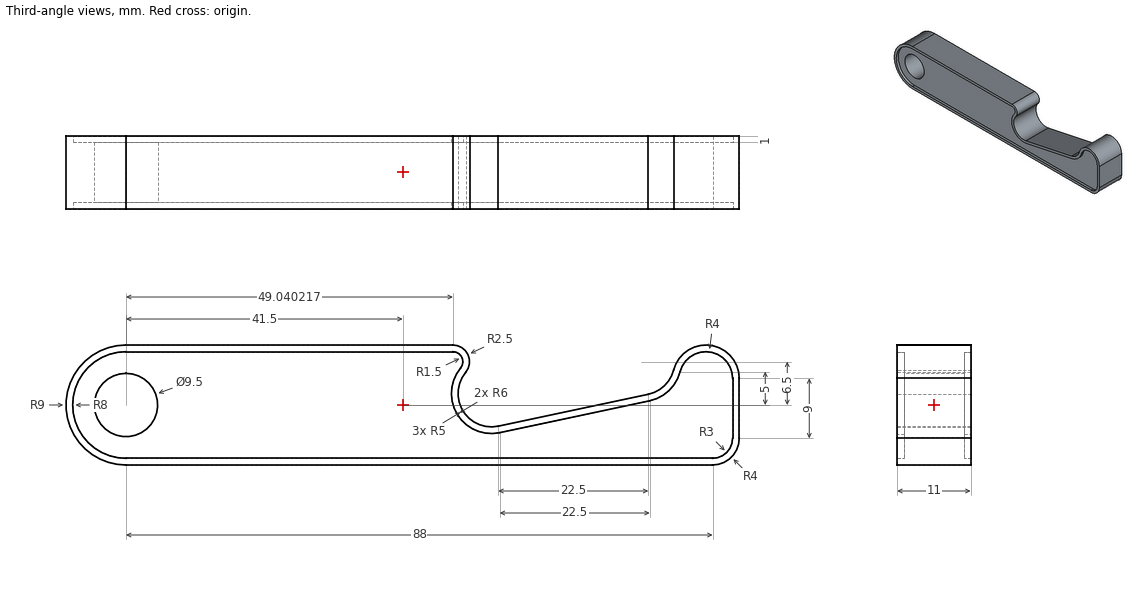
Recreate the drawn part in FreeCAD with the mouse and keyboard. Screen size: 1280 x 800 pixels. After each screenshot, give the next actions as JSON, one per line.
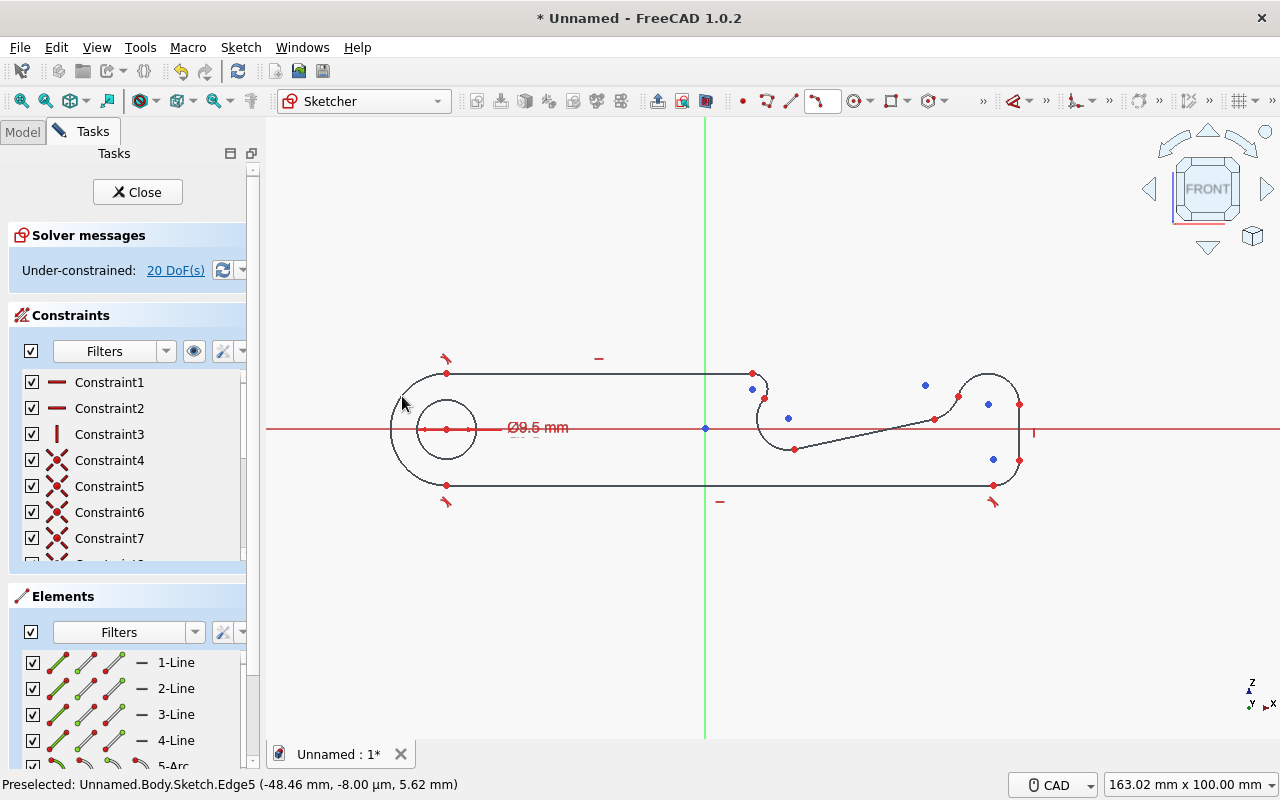
{"action": "left_click", "coordinate": [538, 374]}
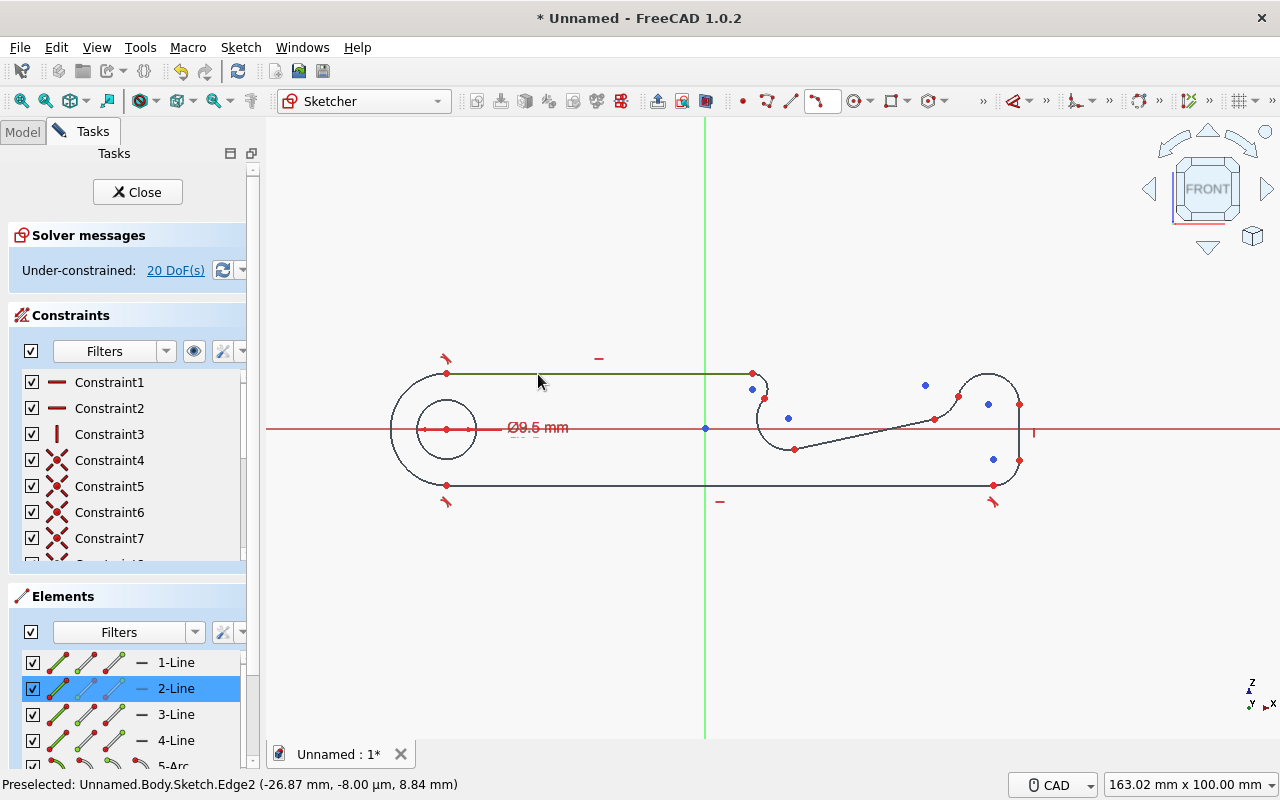
{"action": "scroll", "coordinate": [768, 389], "scroll_direction": "up", "scroll_amount": 2}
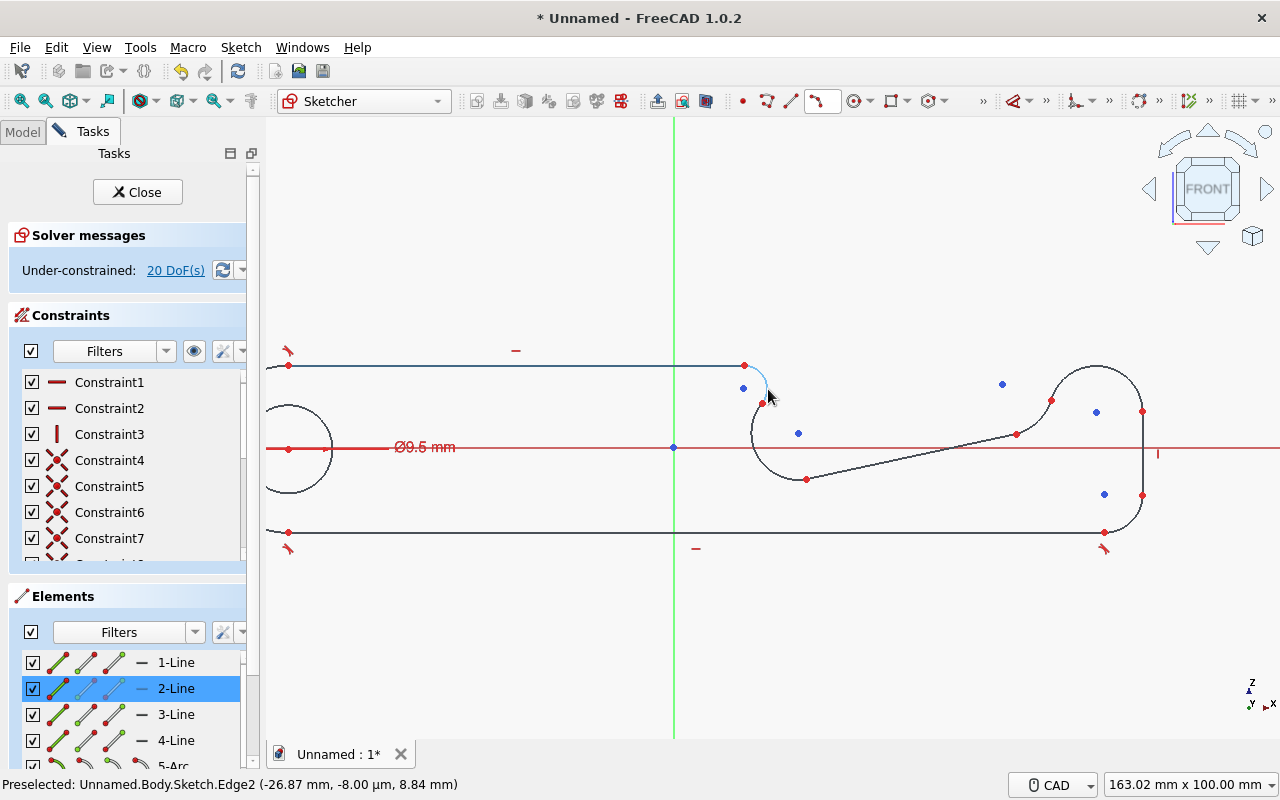
{"action": "left_click", "coordinate": [767, 389]}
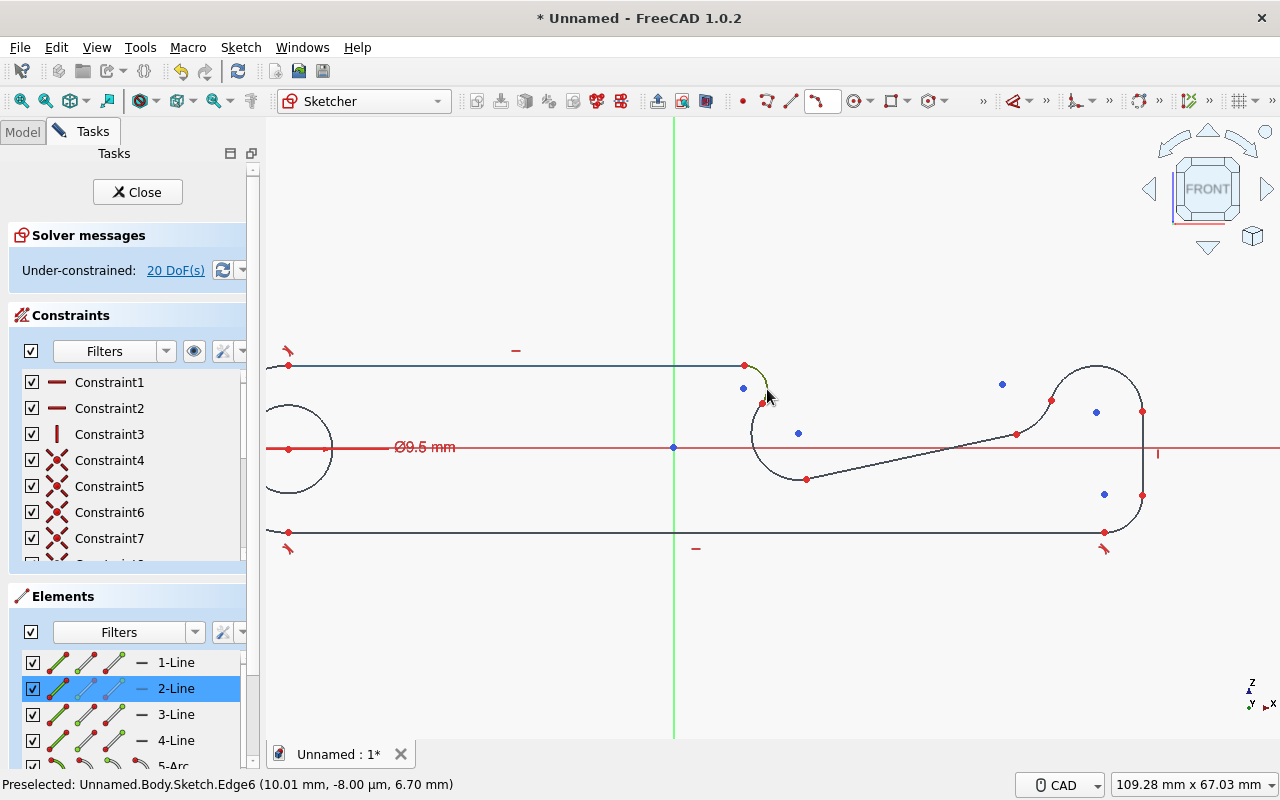
{"action": "key", "text": "t"}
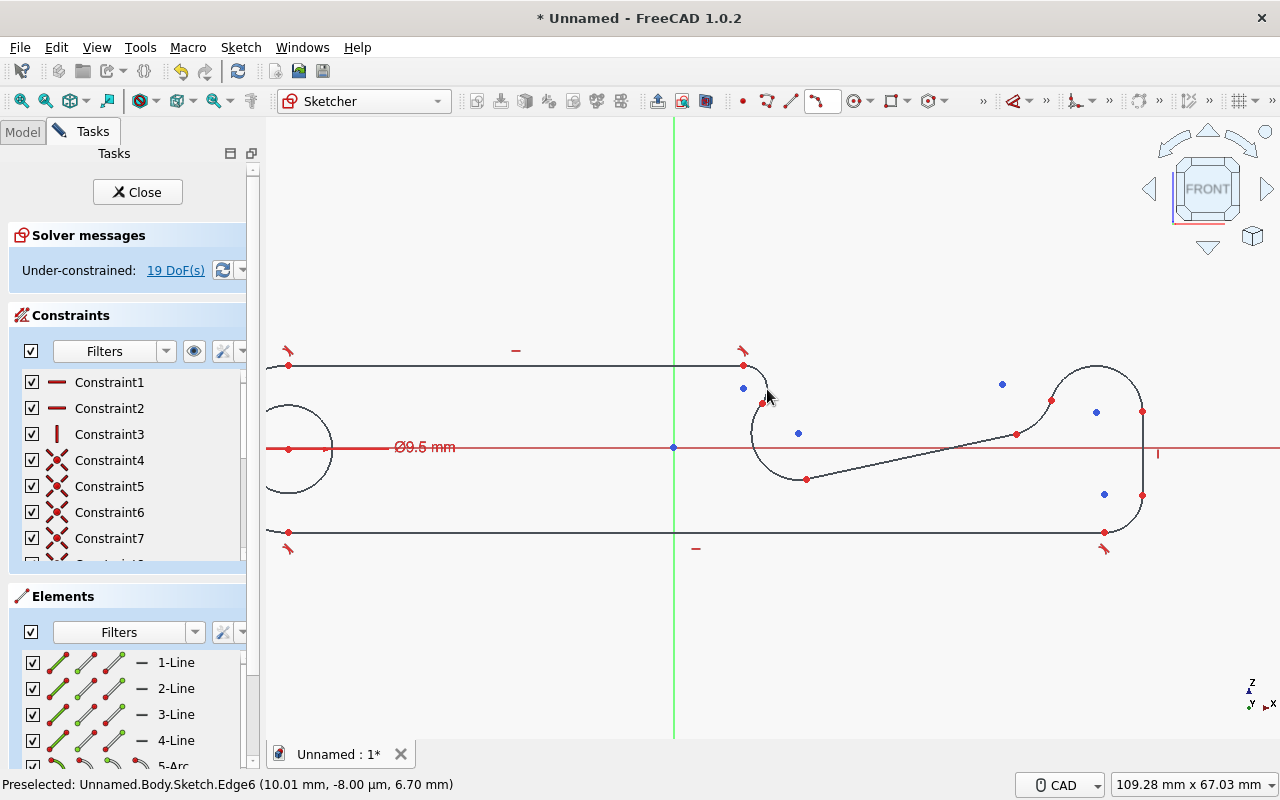
{"action": "left_click", "coordinate": [870, 466]}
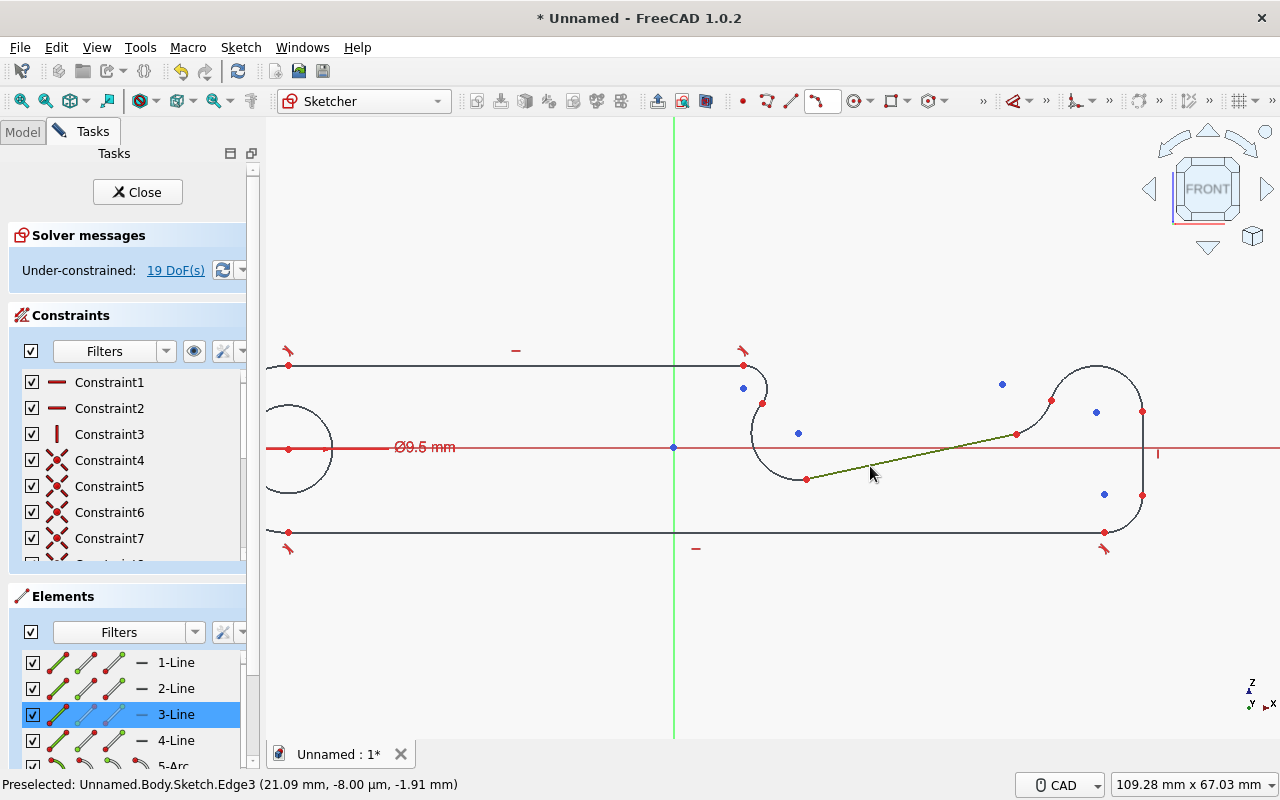
{"action": "left_click", "coordinate": [751, 435]}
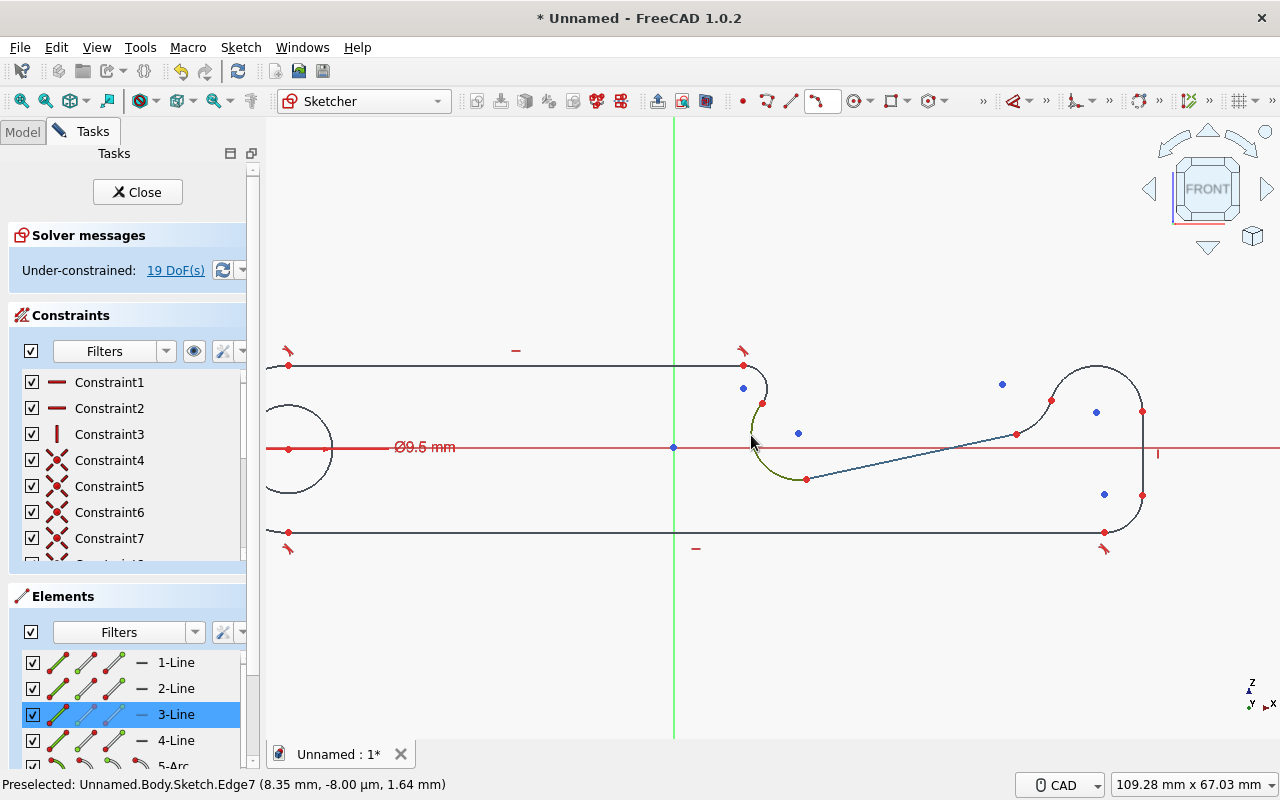
{"action": "key", "text": "t"}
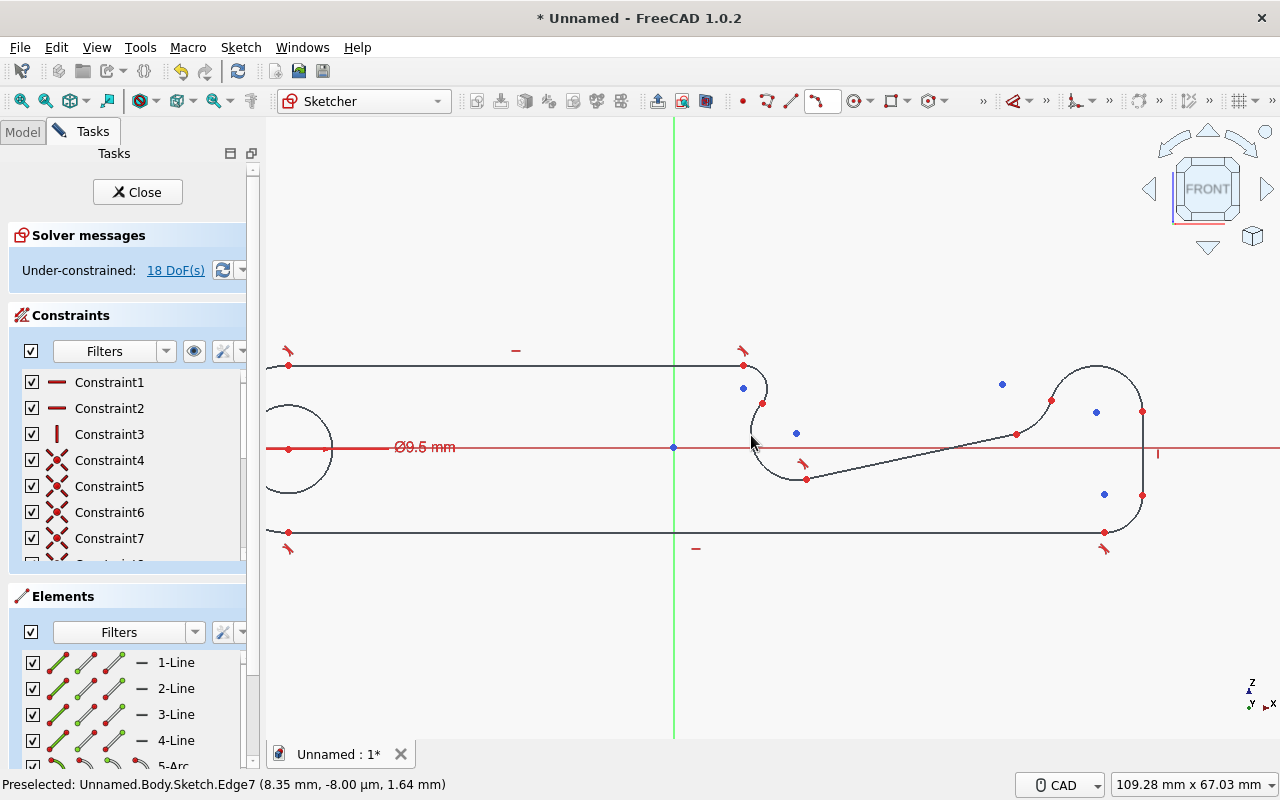
{"action": "left_click", "coordinate": [870, 466]}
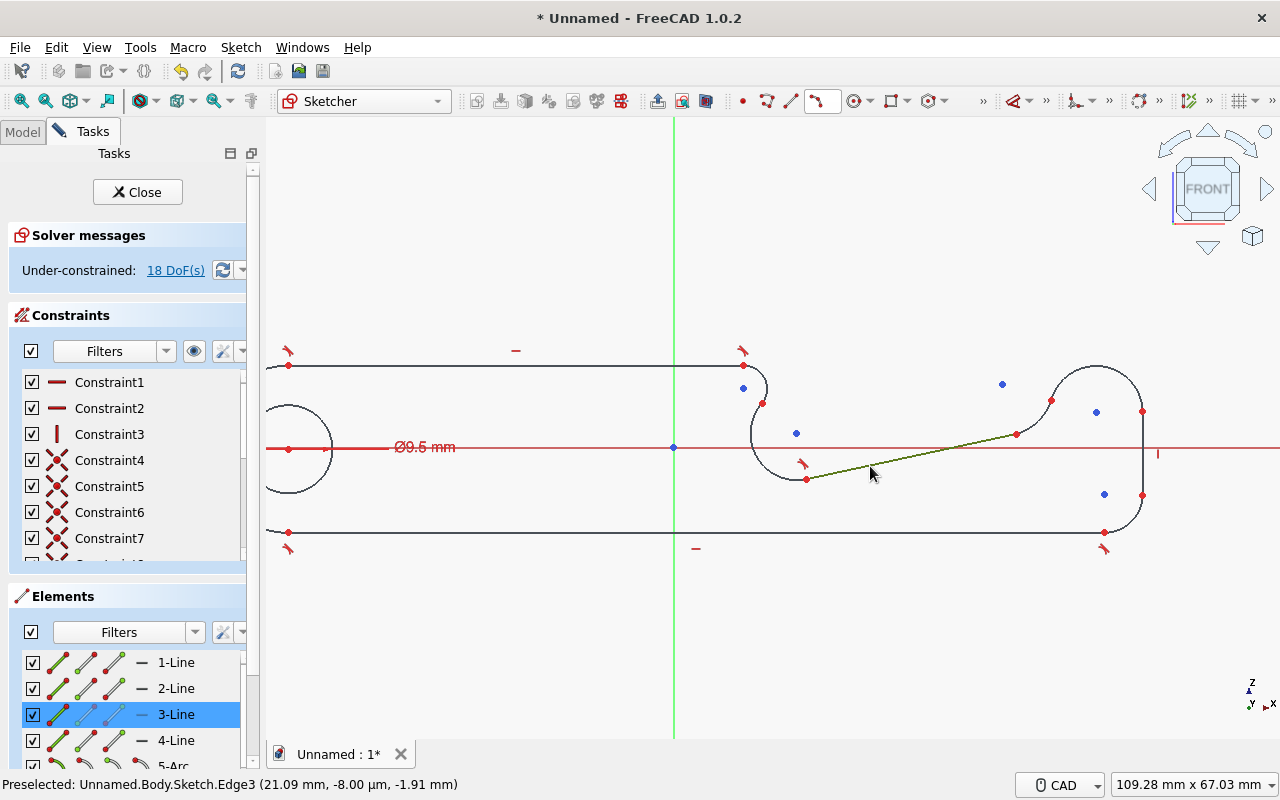
{"action": "left_click", "coordinate": [1030, 428]}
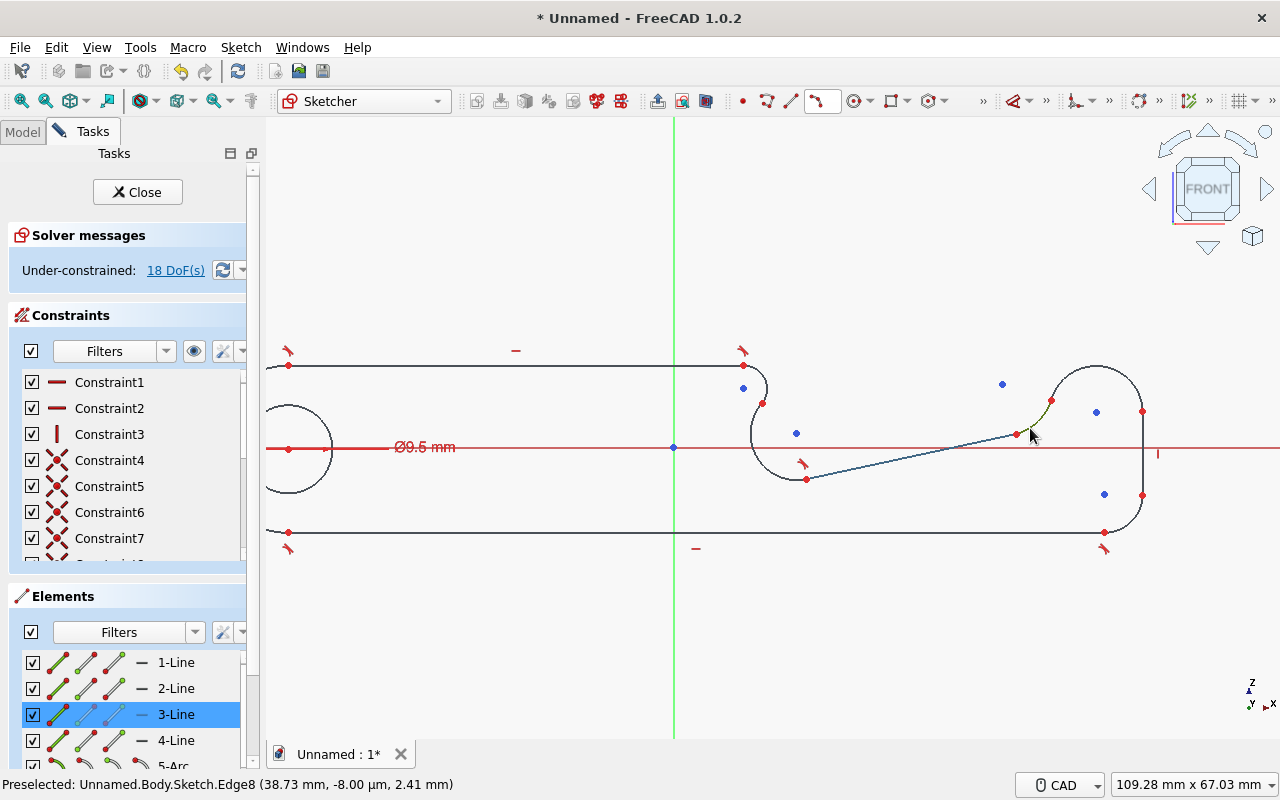
{"action": "key", "text": "t"}